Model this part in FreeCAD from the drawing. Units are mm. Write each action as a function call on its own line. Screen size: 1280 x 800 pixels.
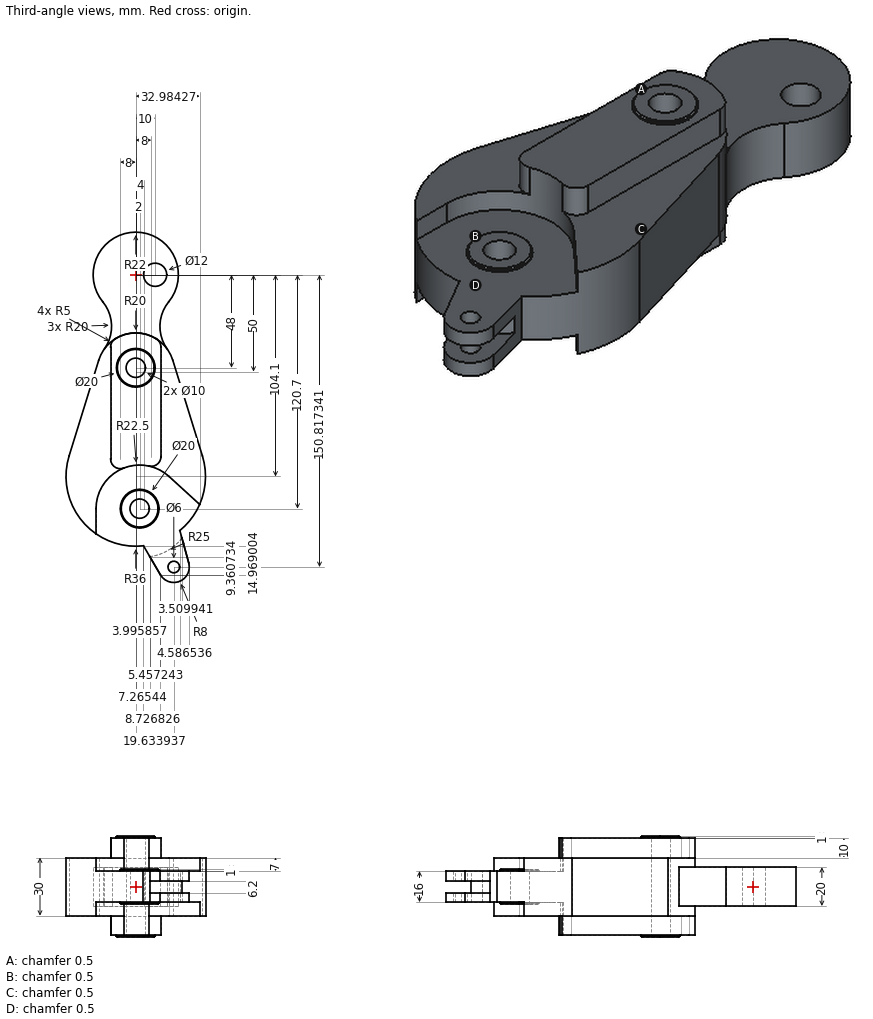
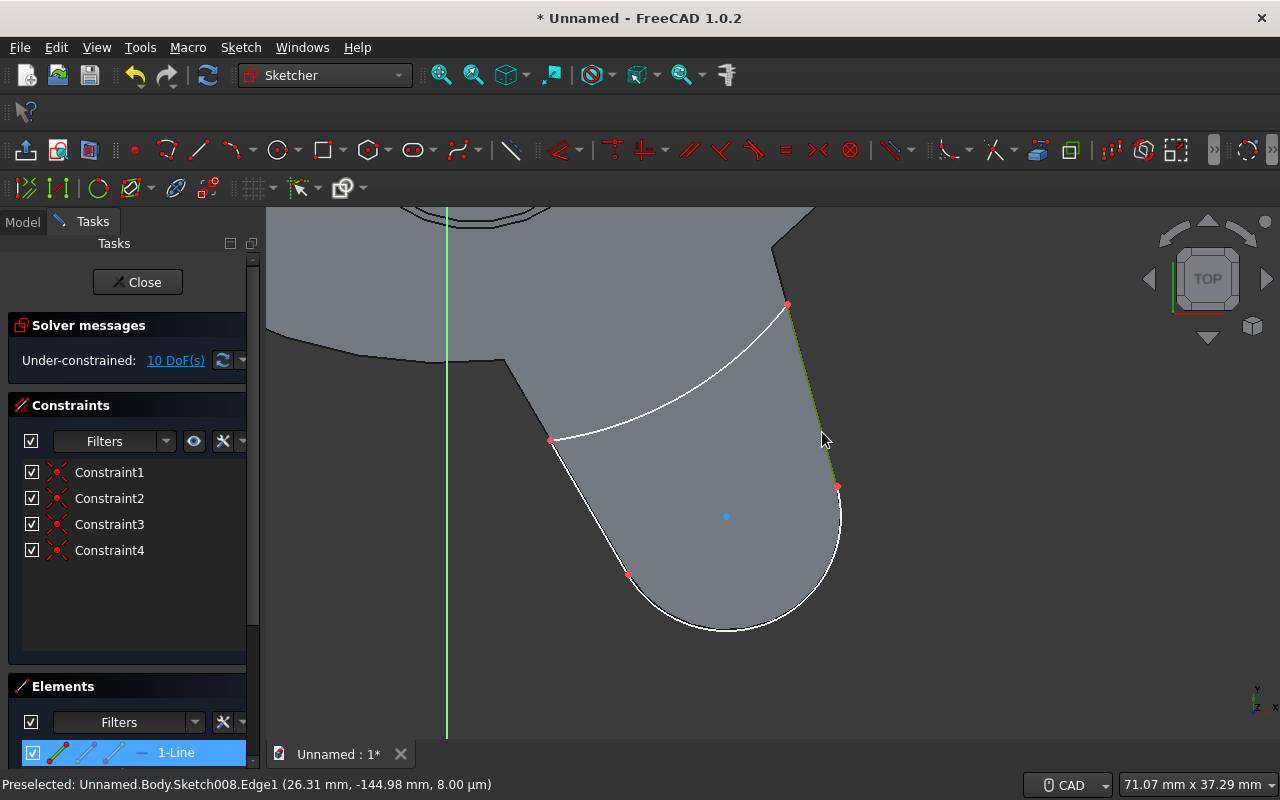
click(707, 629)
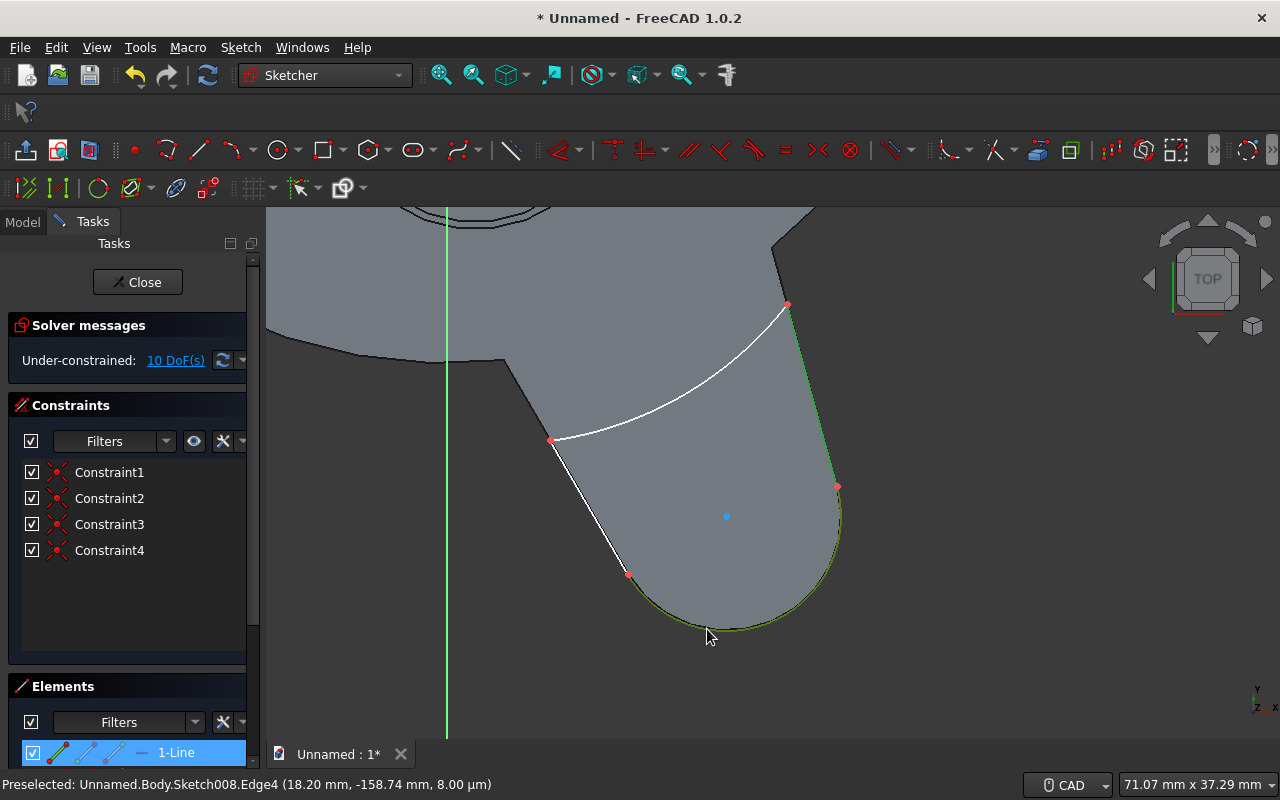
click(754, 150)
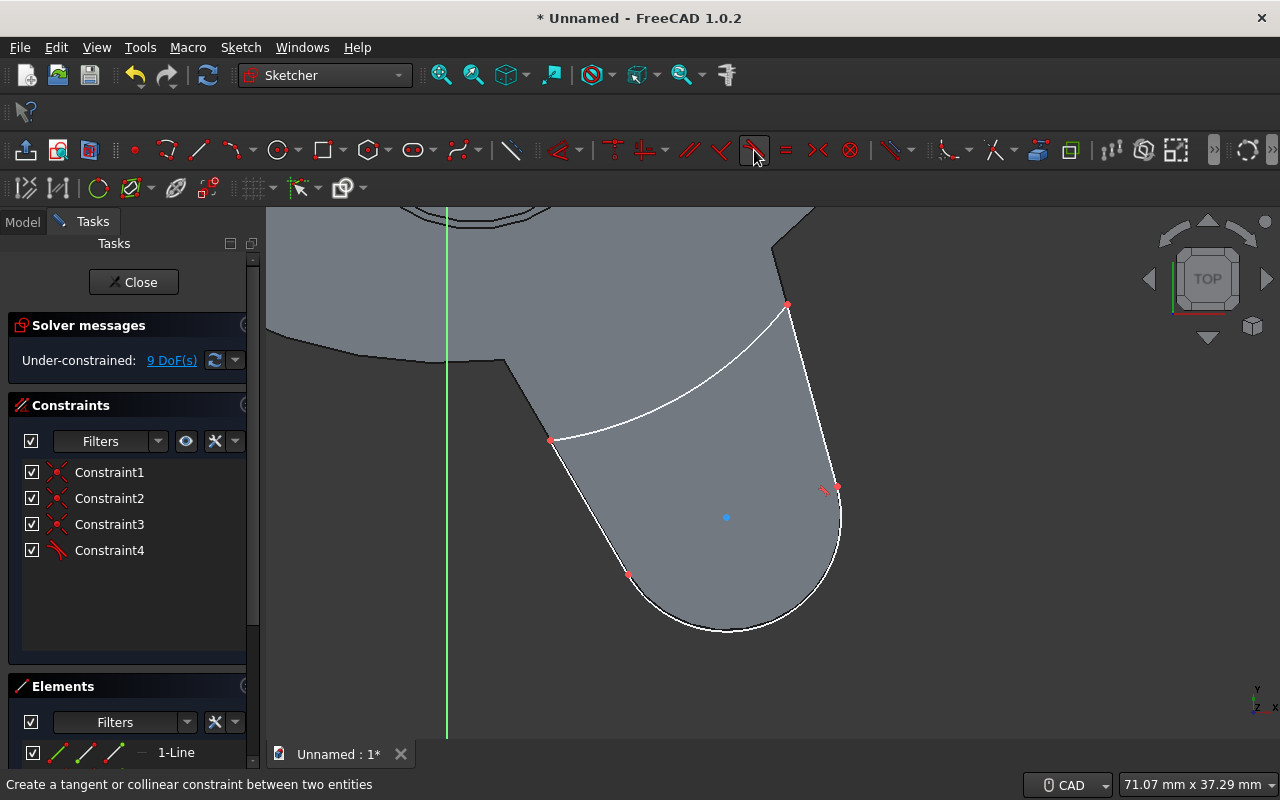
click(573, 481)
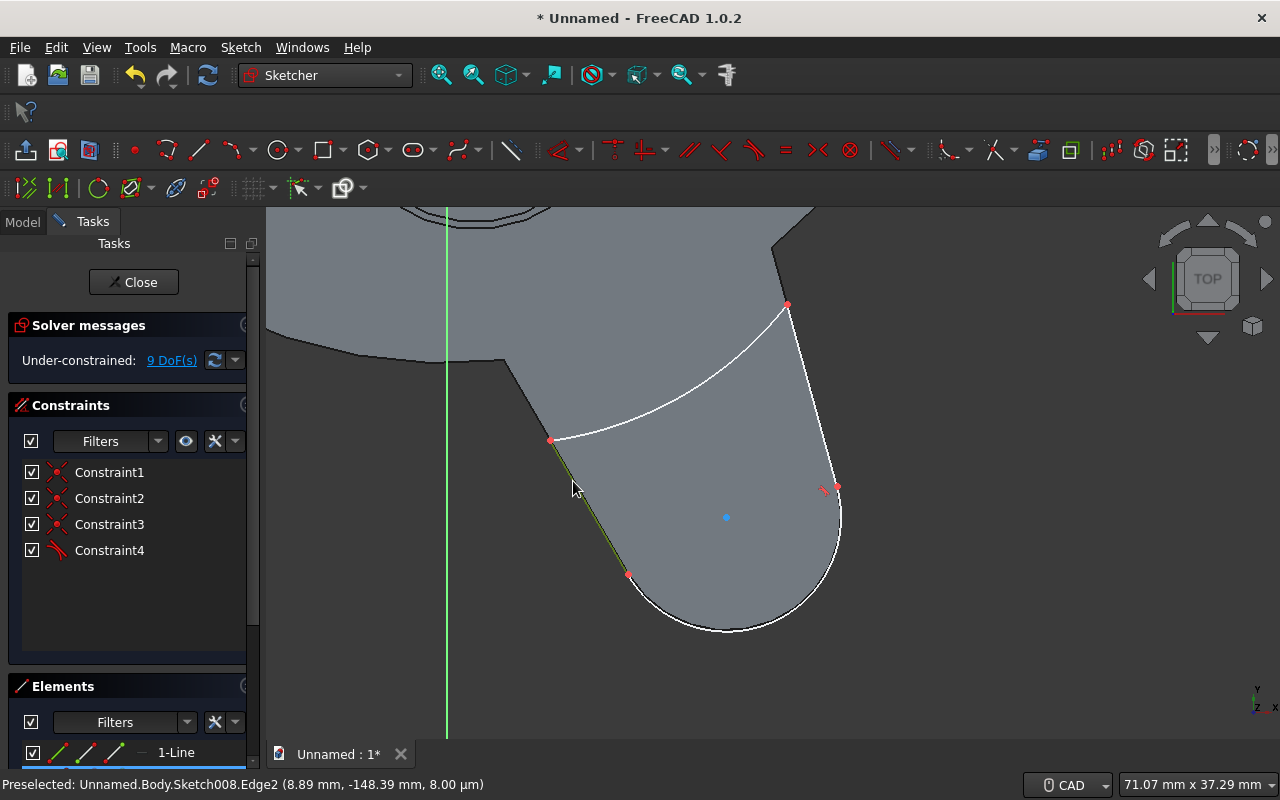
click(707, 630)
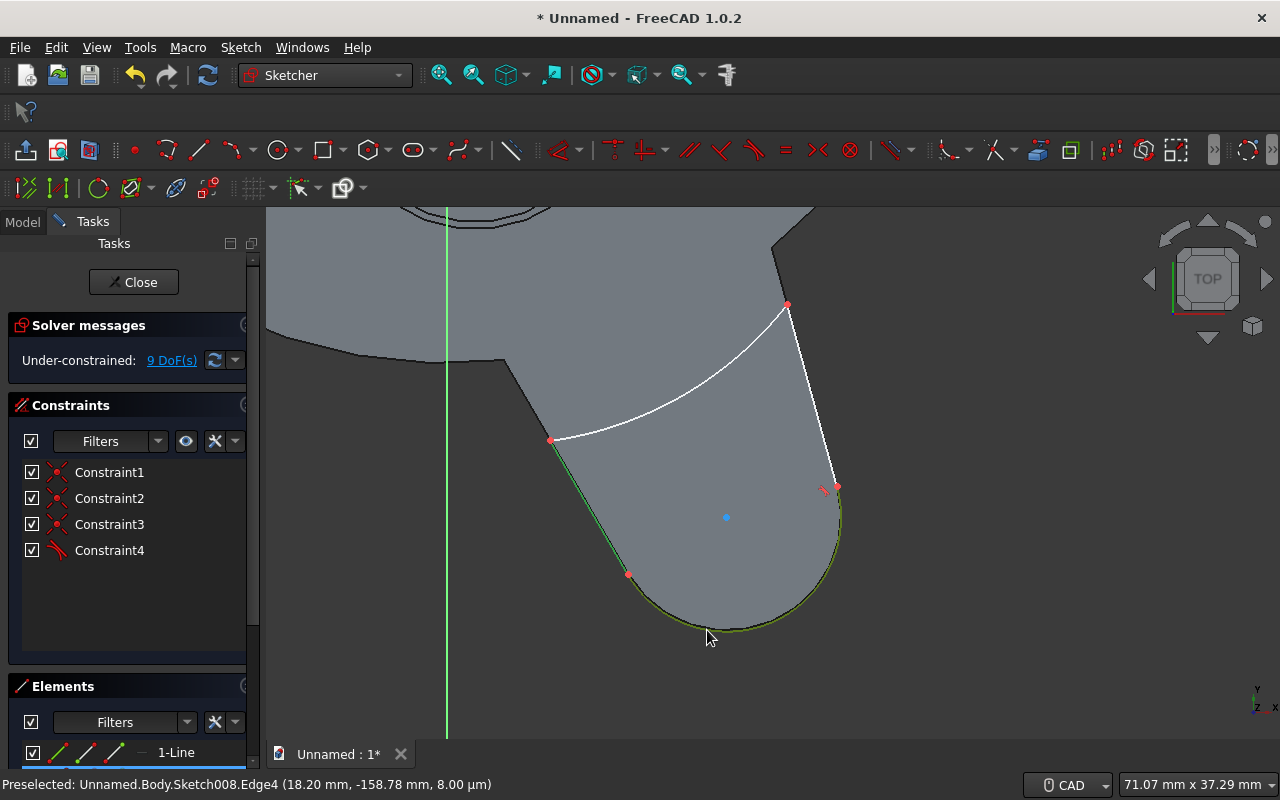
click(754, 150)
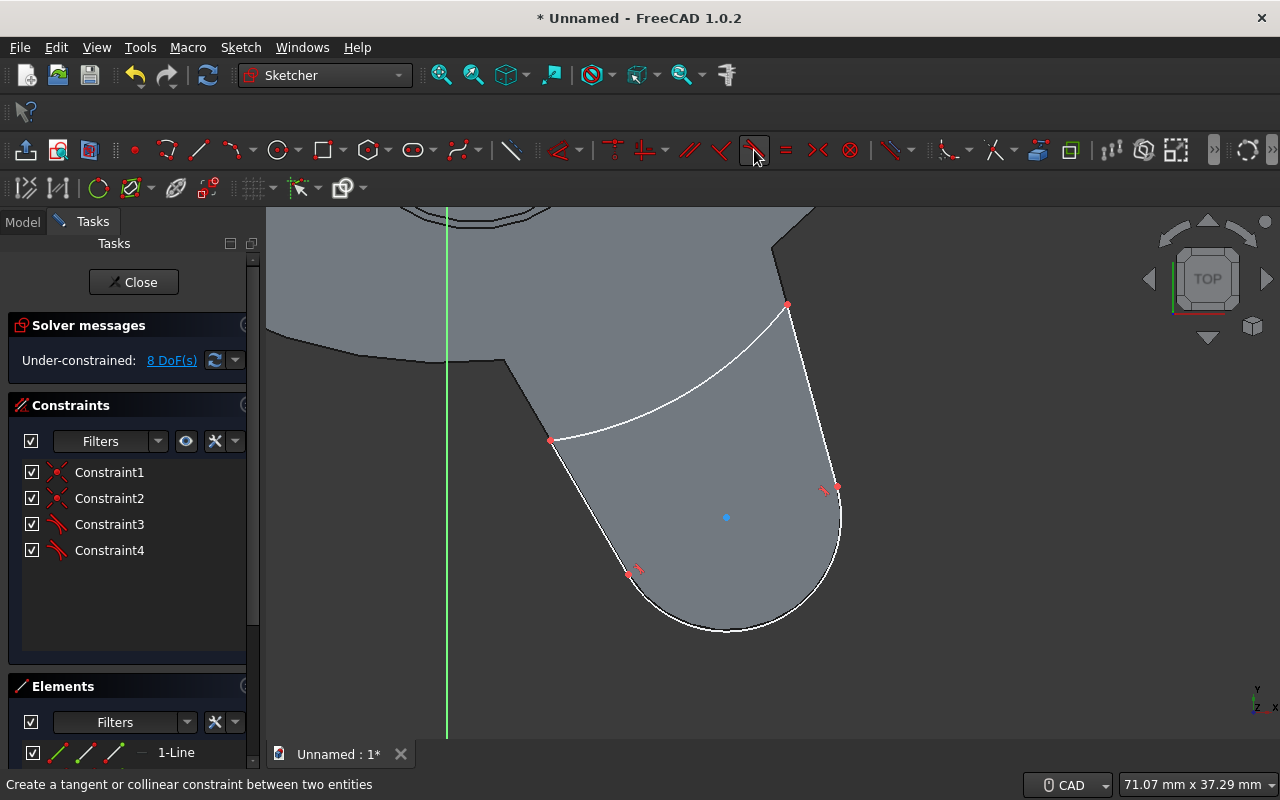
click(558, 150)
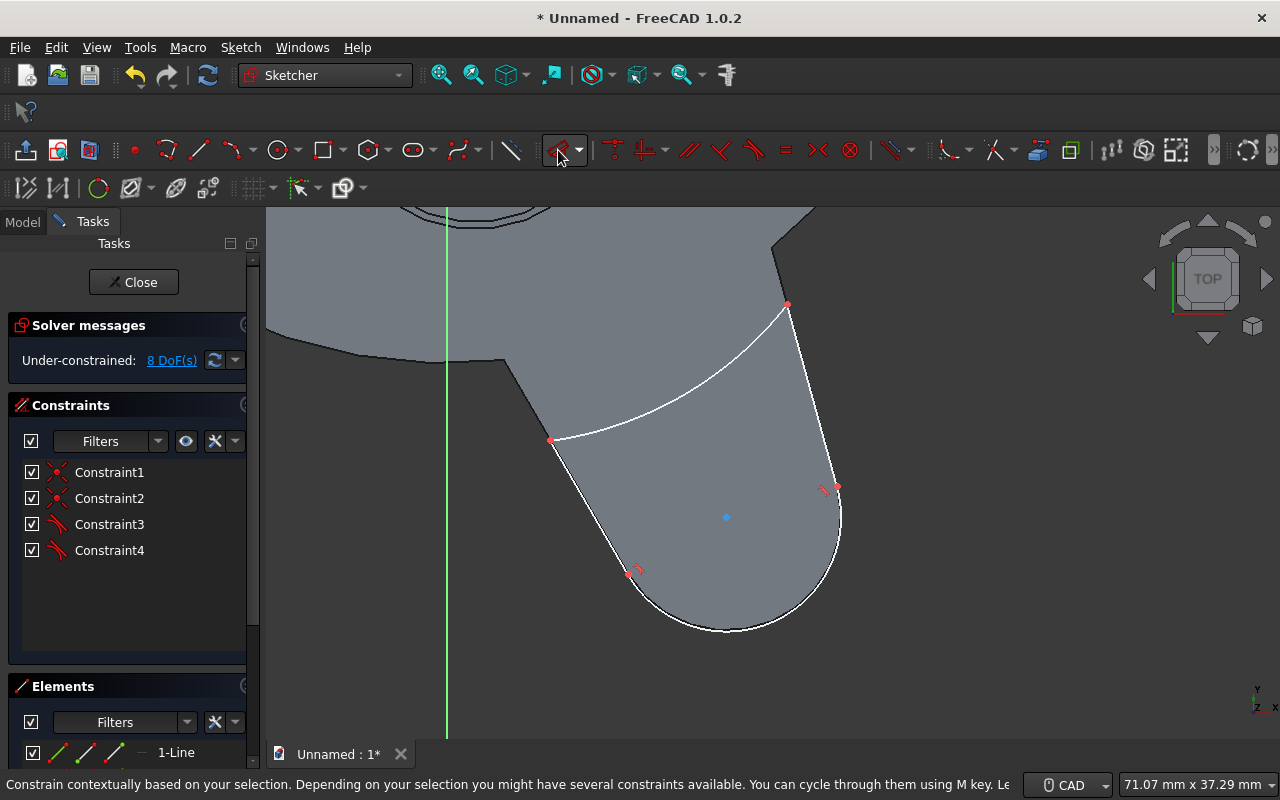
click(631, 420)
click(642, 450)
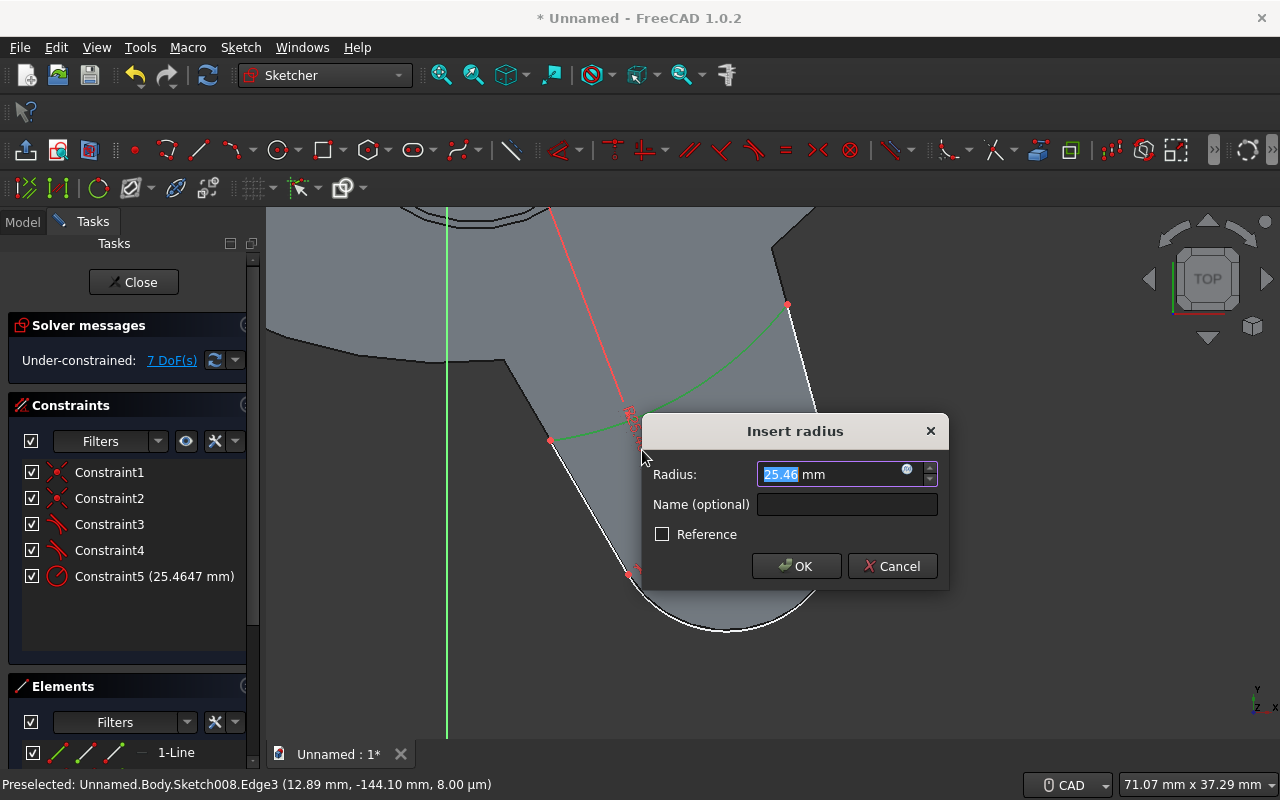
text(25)
key(Return)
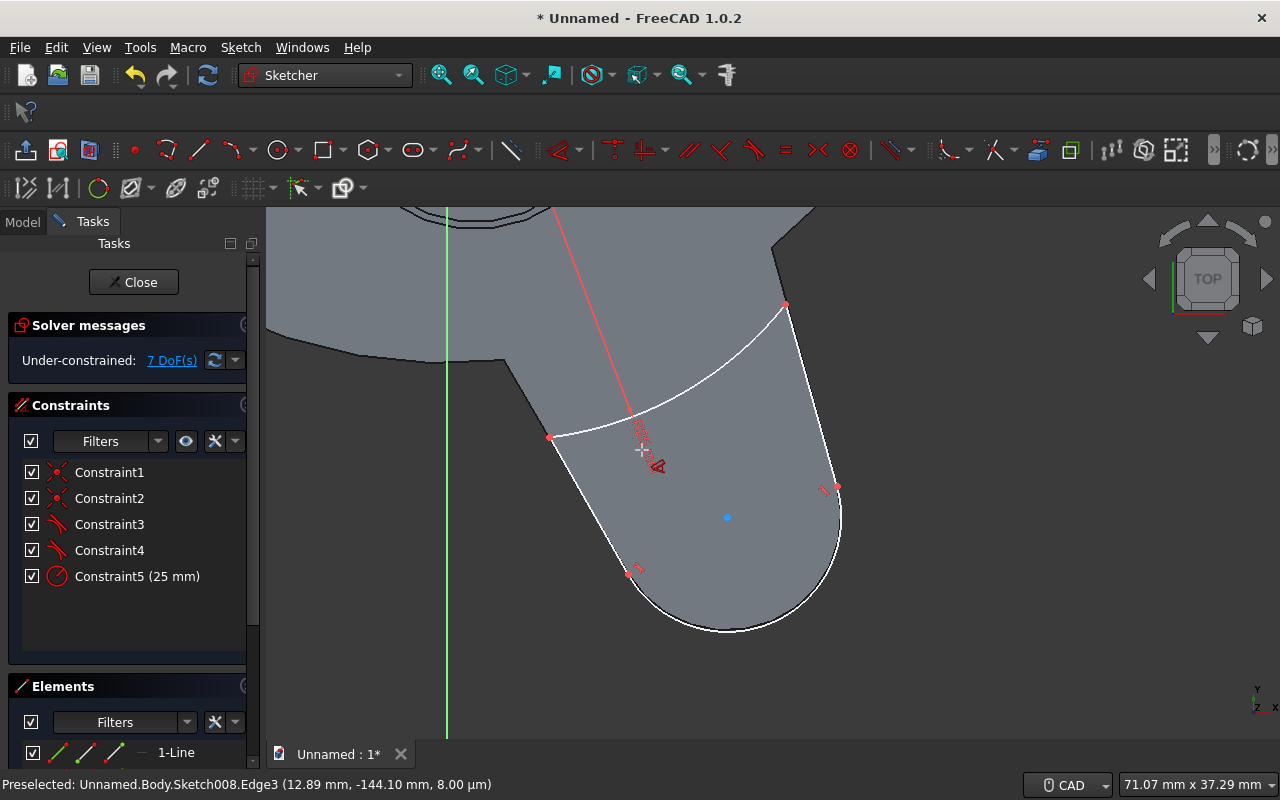
click(706, 630)
click(700, 661)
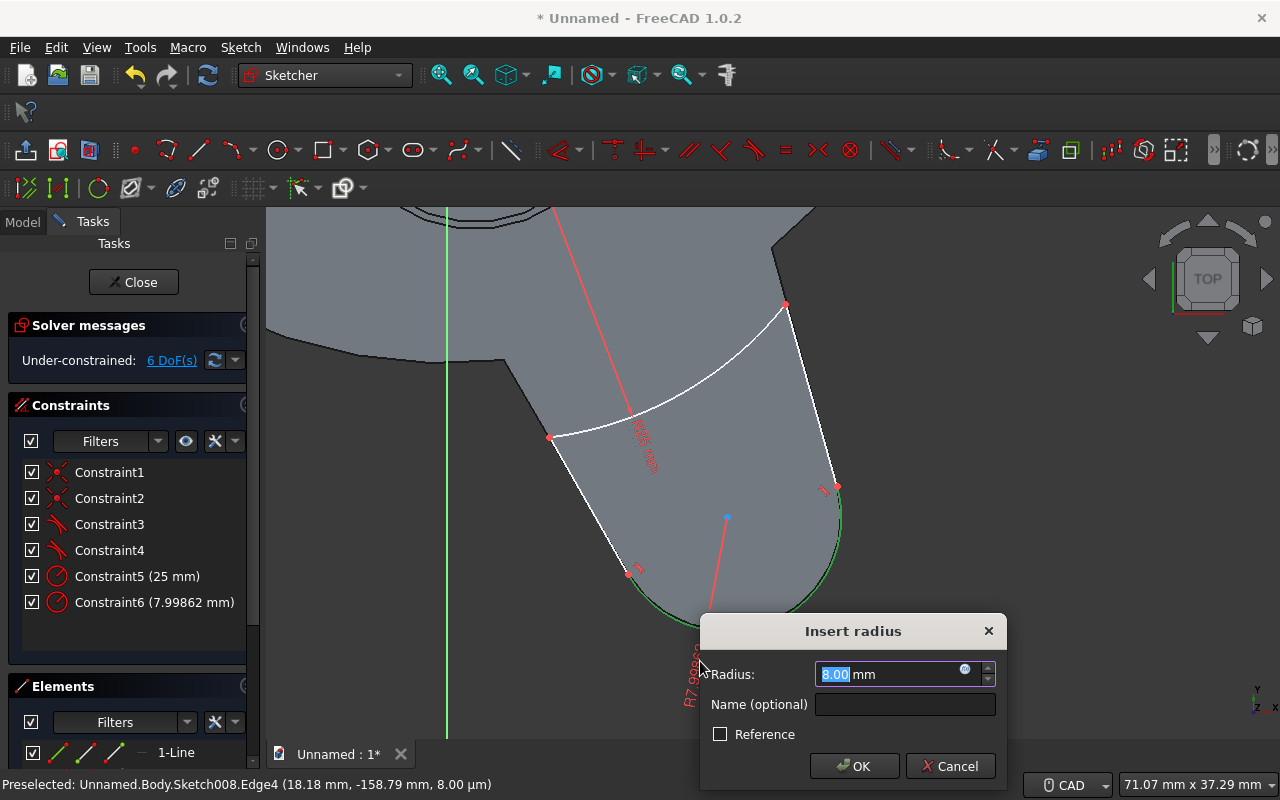
text(8)
key(Return)